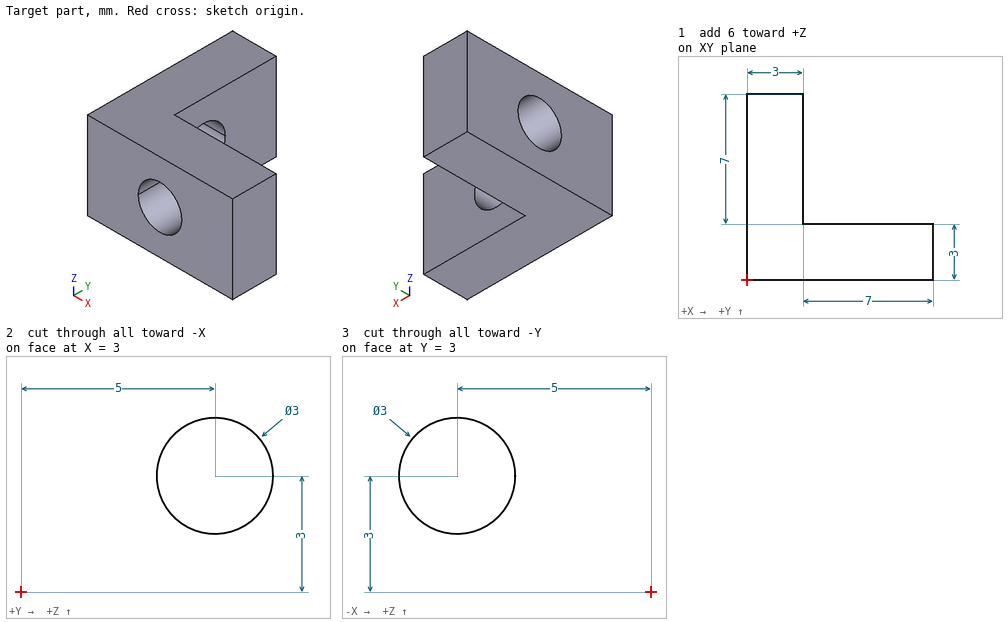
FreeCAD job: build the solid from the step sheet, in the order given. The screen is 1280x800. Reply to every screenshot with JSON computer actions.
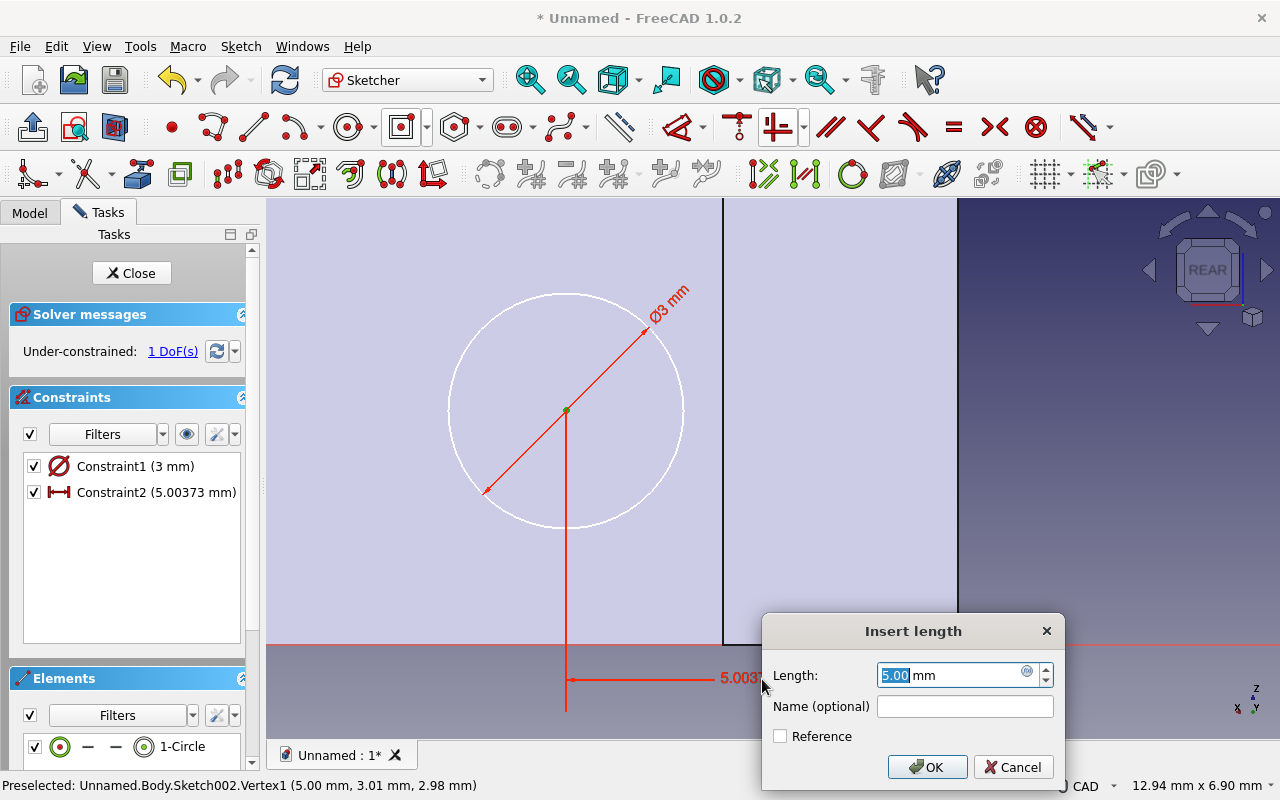
{"action": "type", "text": "5"}
{"action": "key", "text": "Return"}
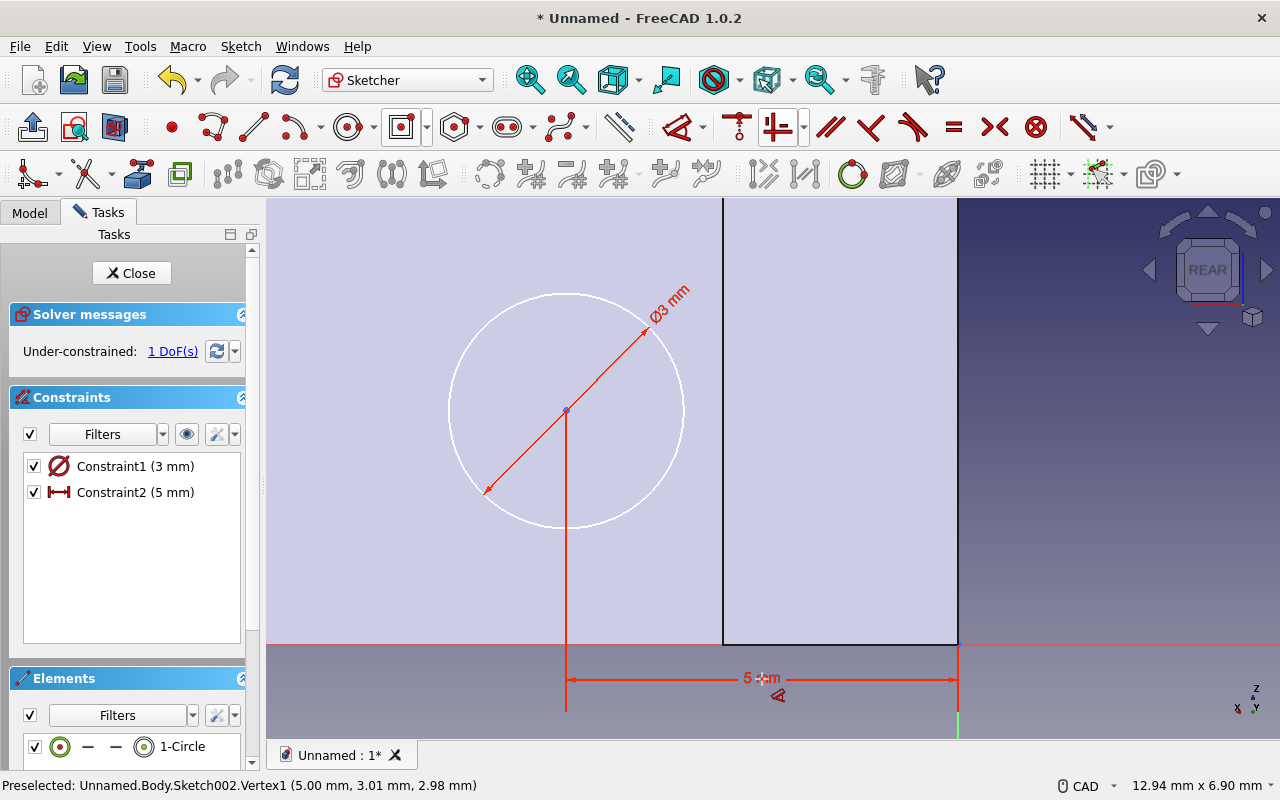
{"action": "left_click", "coordinate": [566, 411]}
{"action": "left_click", "coordinate": [992, 528]}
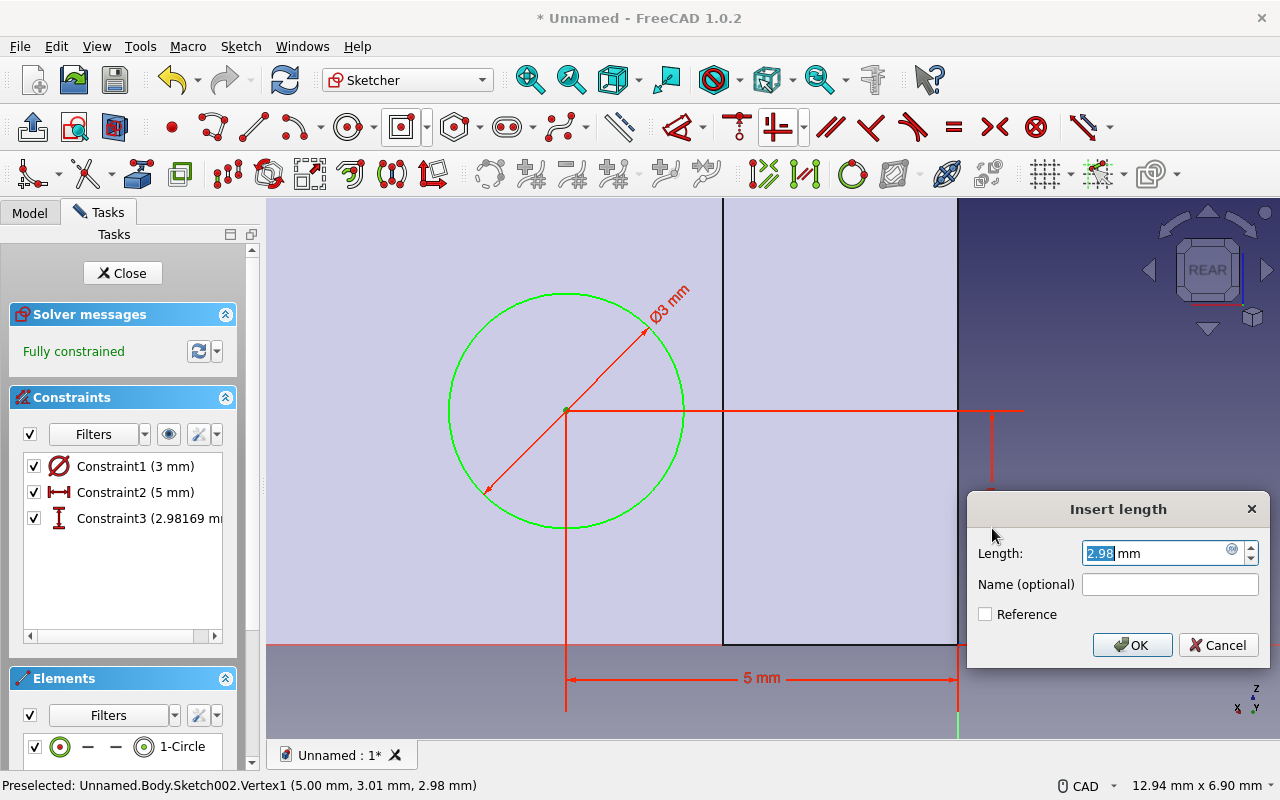
{"action": "type", "text": "3"}
{"action": "key", "text": "Return"}
{"action": "key", "text": "Escape"}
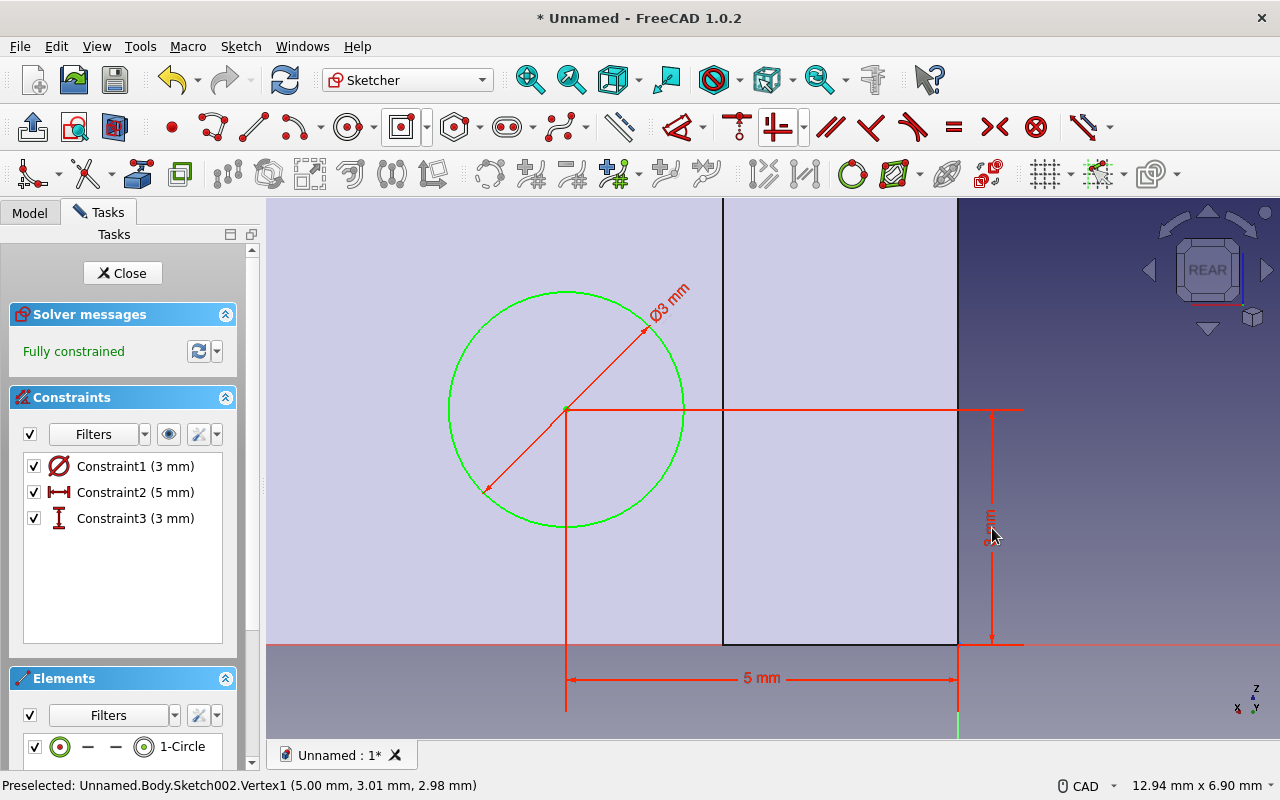
{"action": "left_click", "coordinate": [123, 273]}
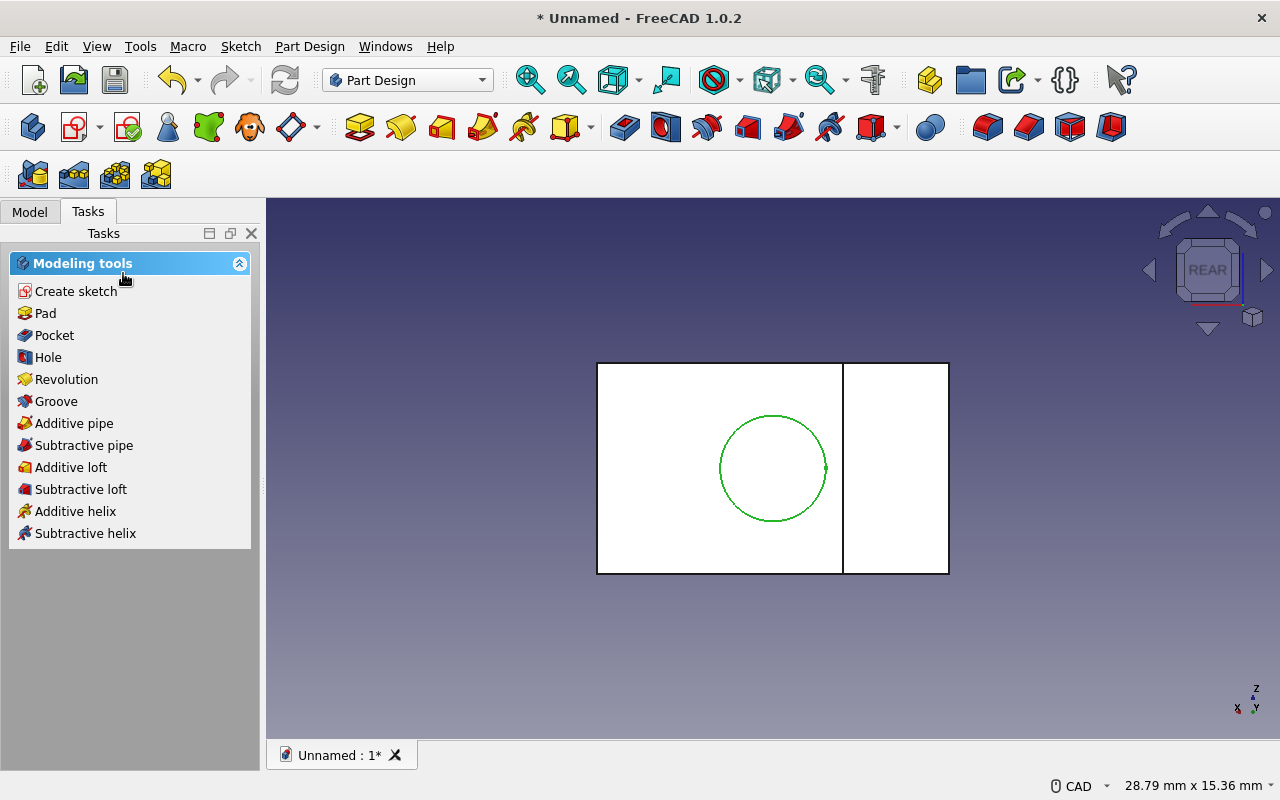
{"action": "left_click", "coordinate": [625, 128]}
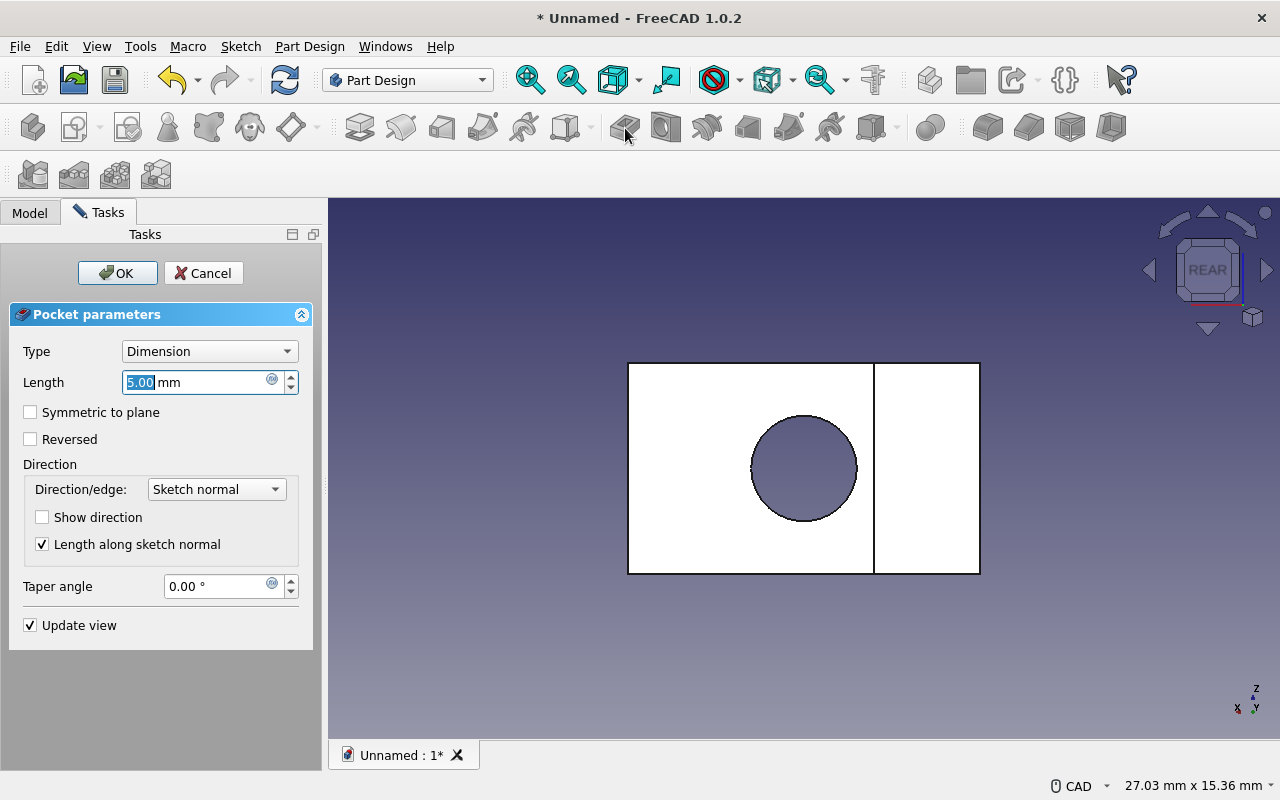
{"action": "left_click", "coordinate": [210, 352]}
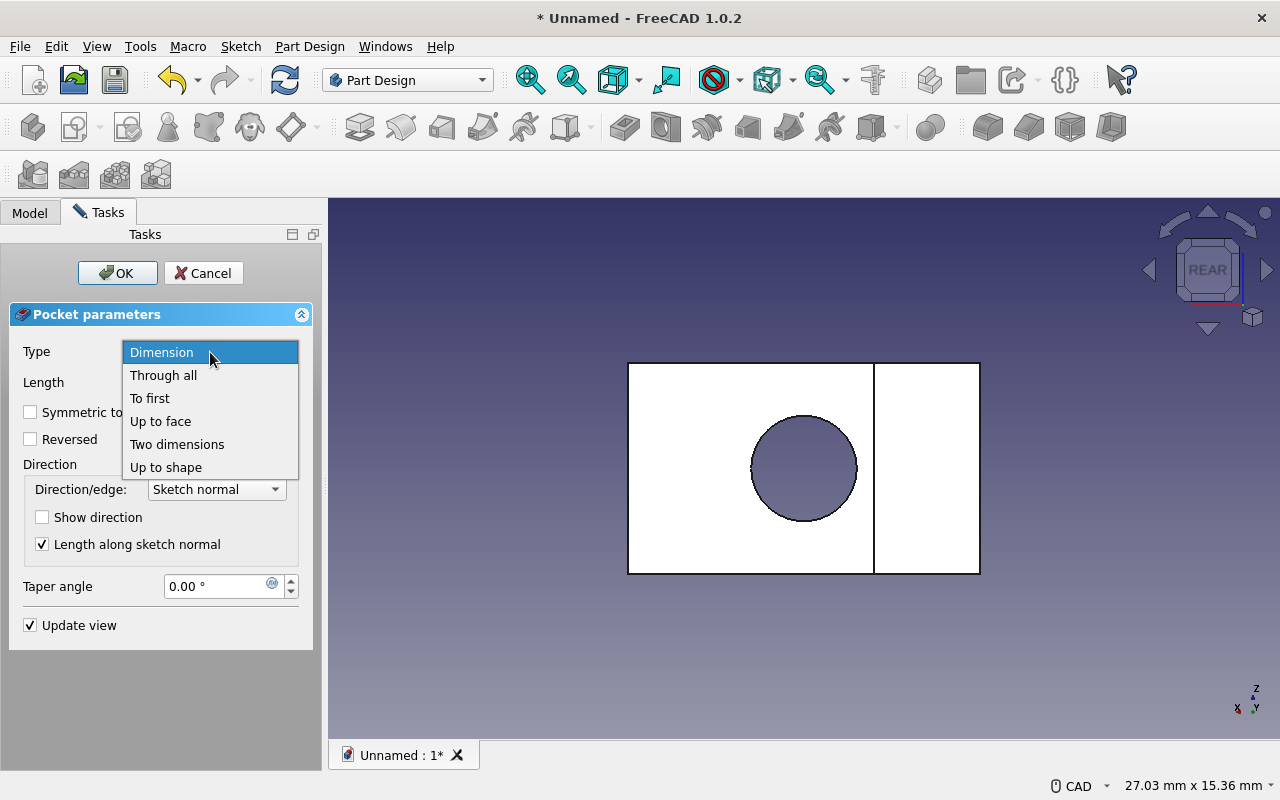
{"action": "left_click", "coordinate": [208, 376]}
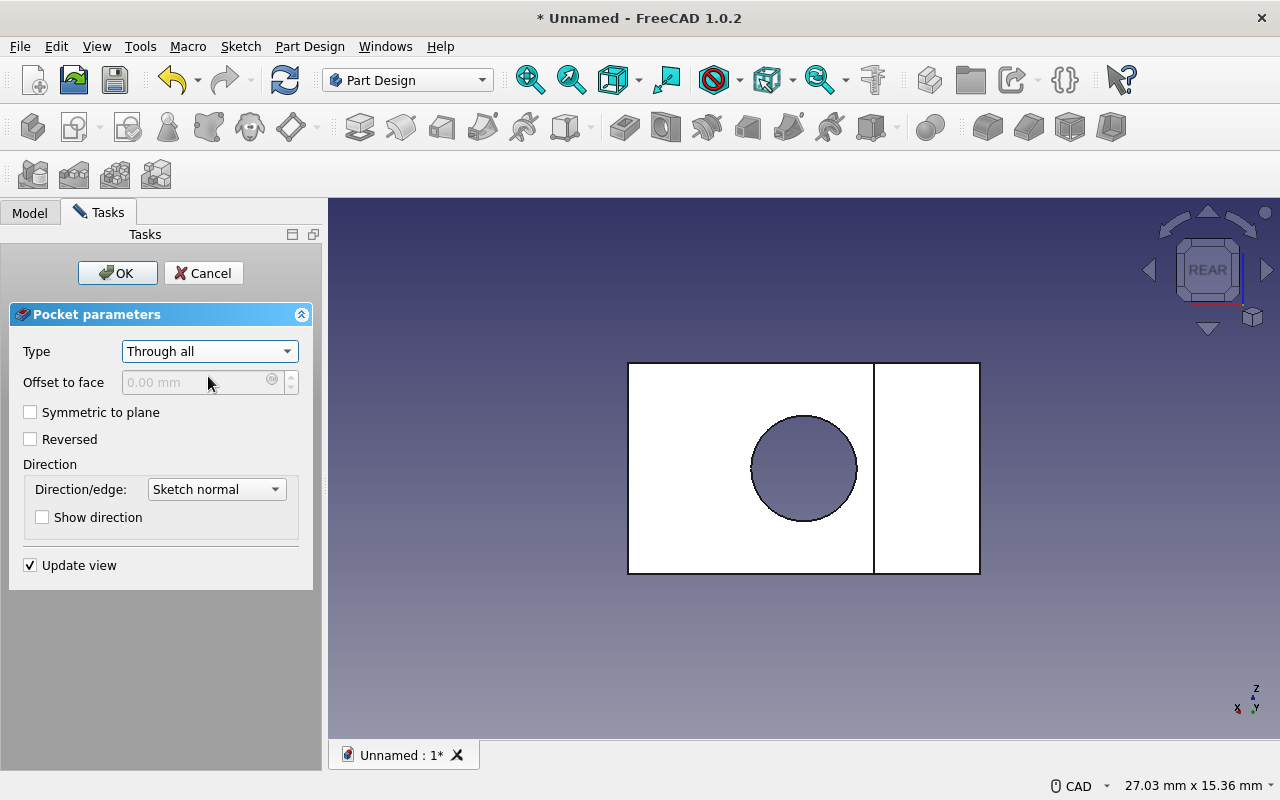
{"action": "left_click", "coordinate": [118, 273]}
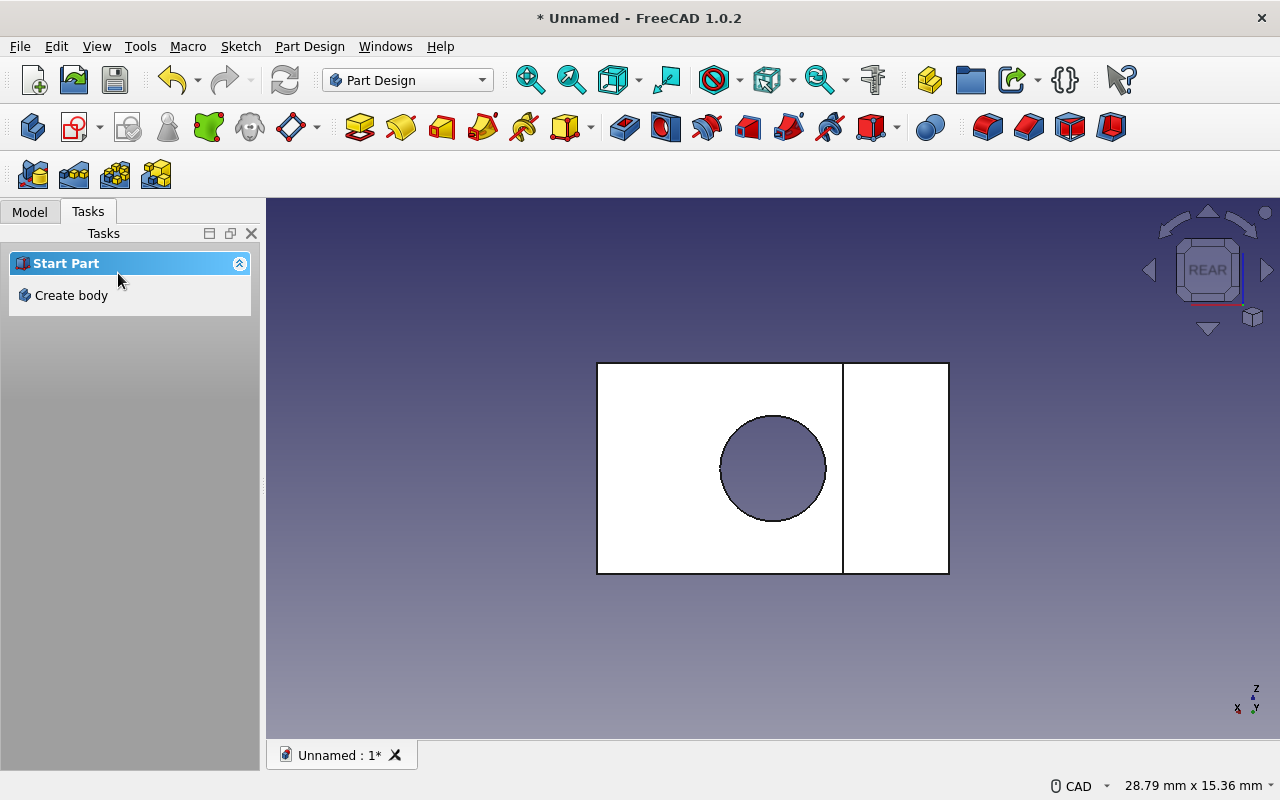
{"action": "key", "text": "0"}